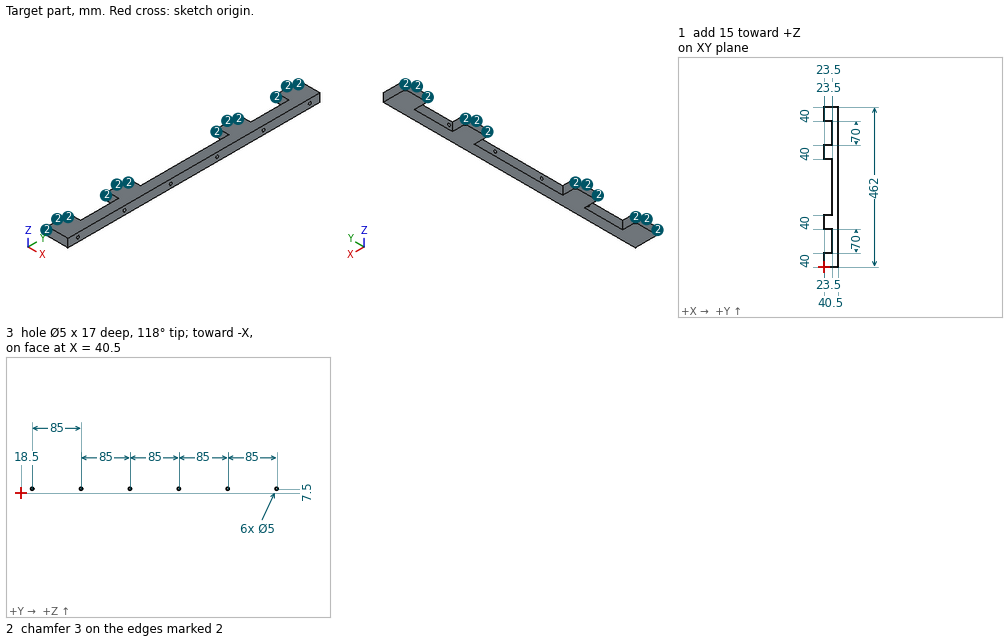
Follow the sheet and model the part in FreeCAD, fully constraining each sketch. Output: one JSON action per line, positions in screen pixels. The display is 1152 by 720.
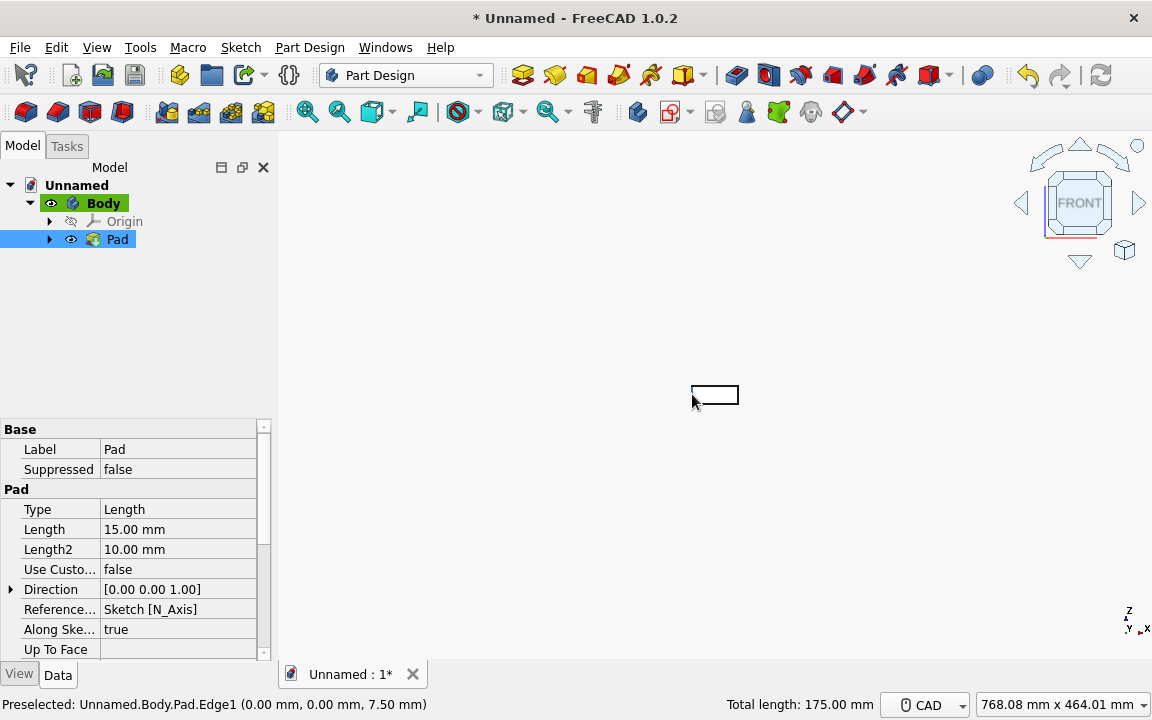
{"action": "scroll", "coordinate": [692, 394], "scroll_direction": "up", "scroll_amount": 5}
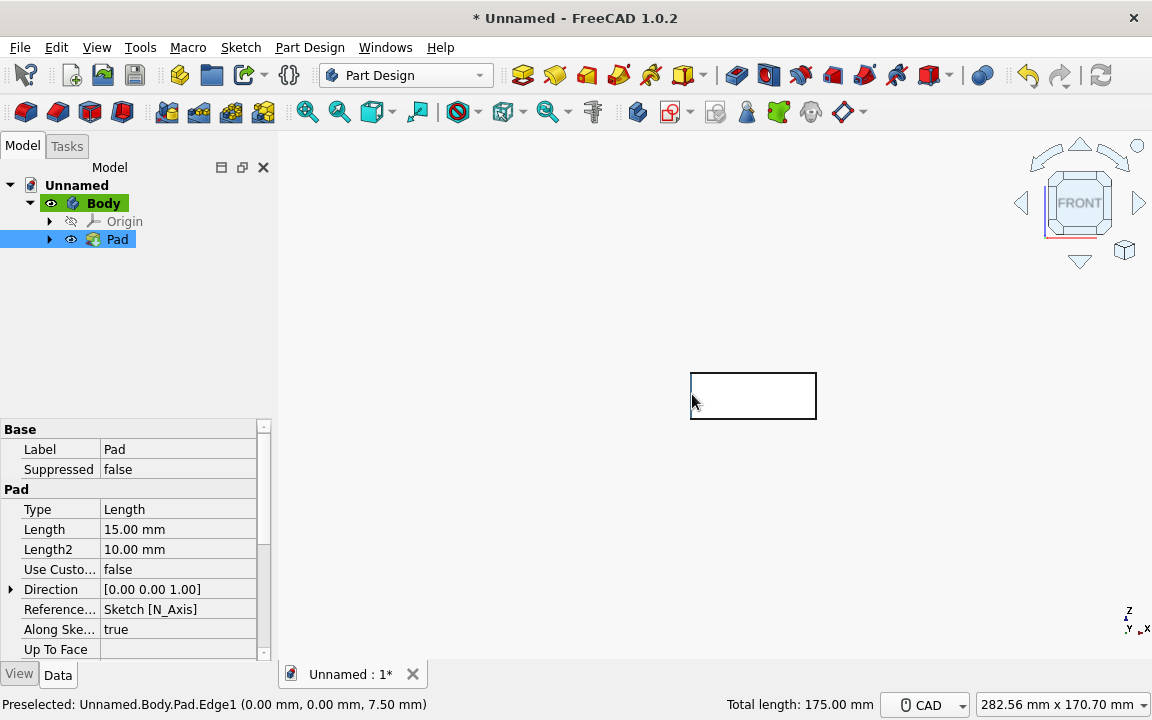
{"action": "left_click", "coordinate": [308, 112]}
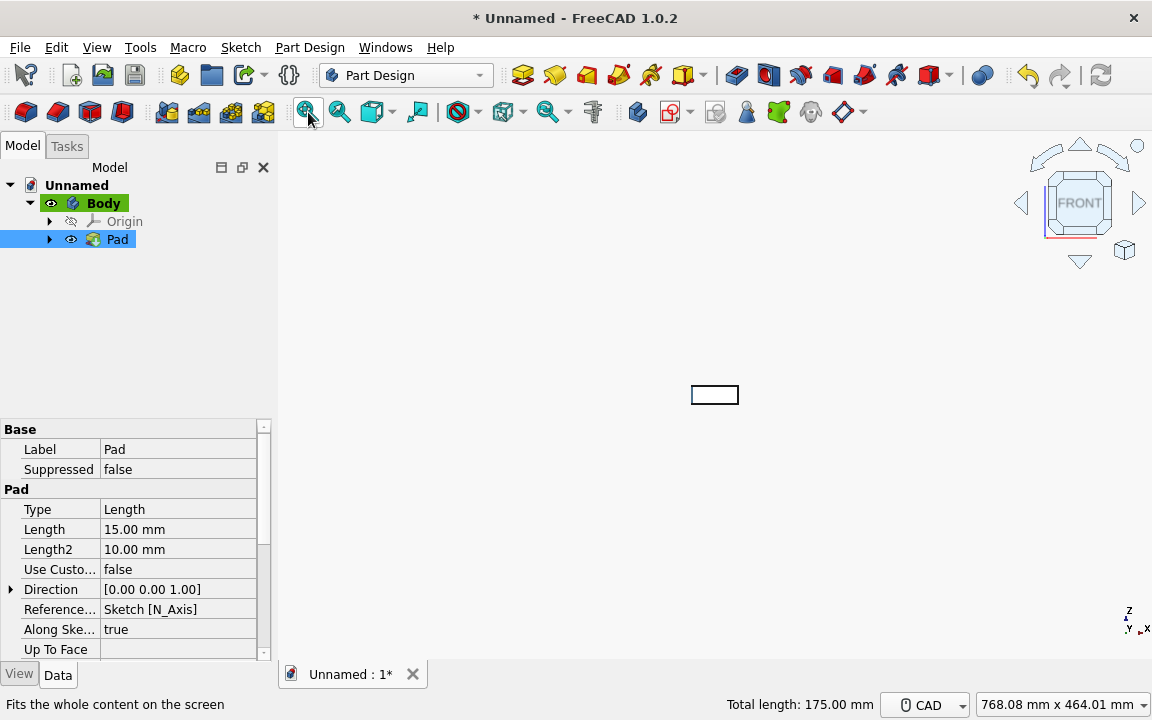
{"action": "key", "text": "3"}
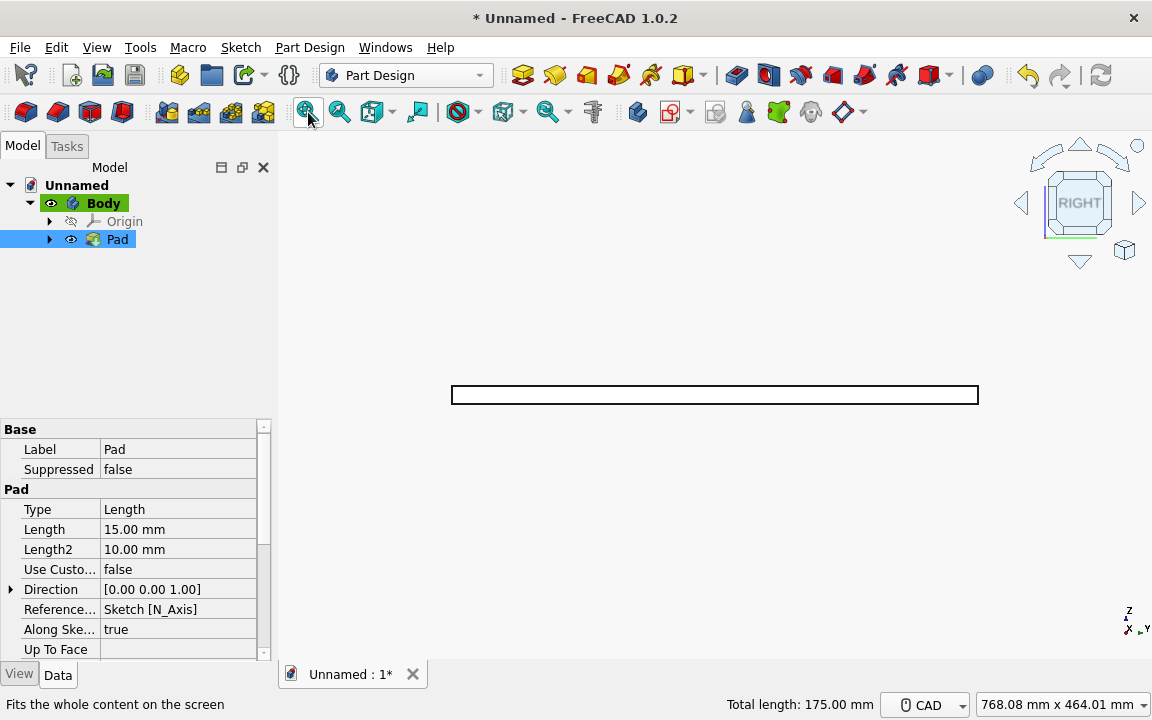
{"action": "scroll", "coordinate": [577, 394], "scroll_direction": "up", "scroll_amount": 5}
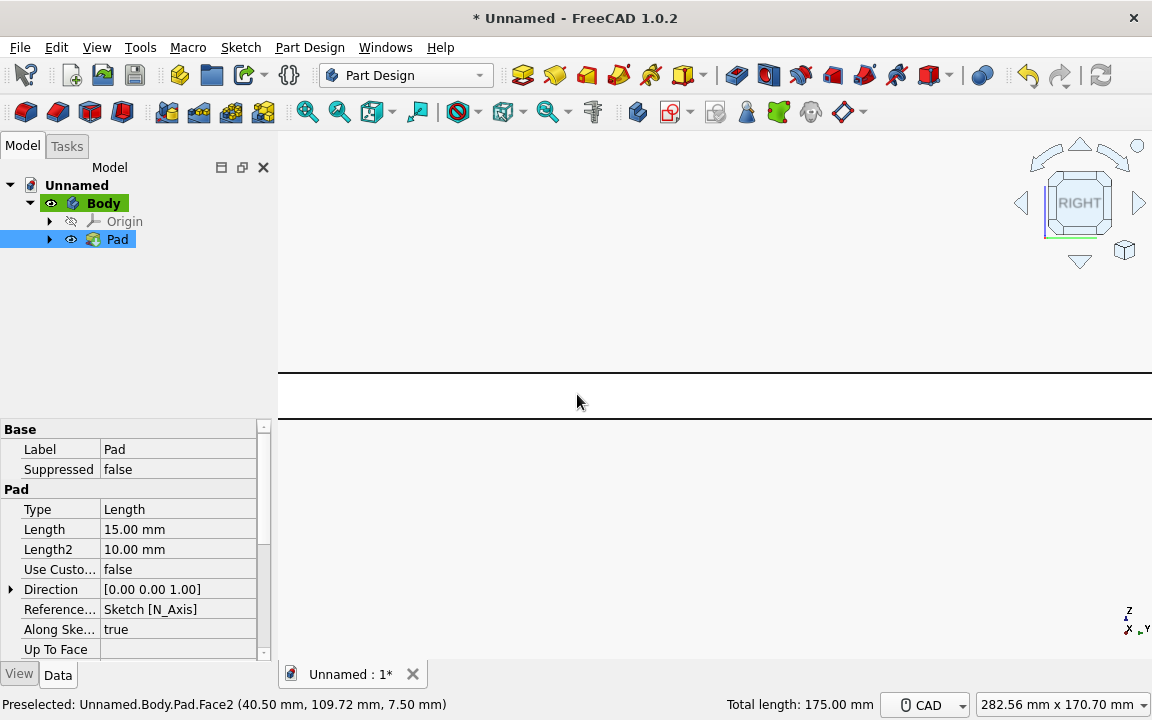
{"action": "left_click", "coordinate": [308, 112]}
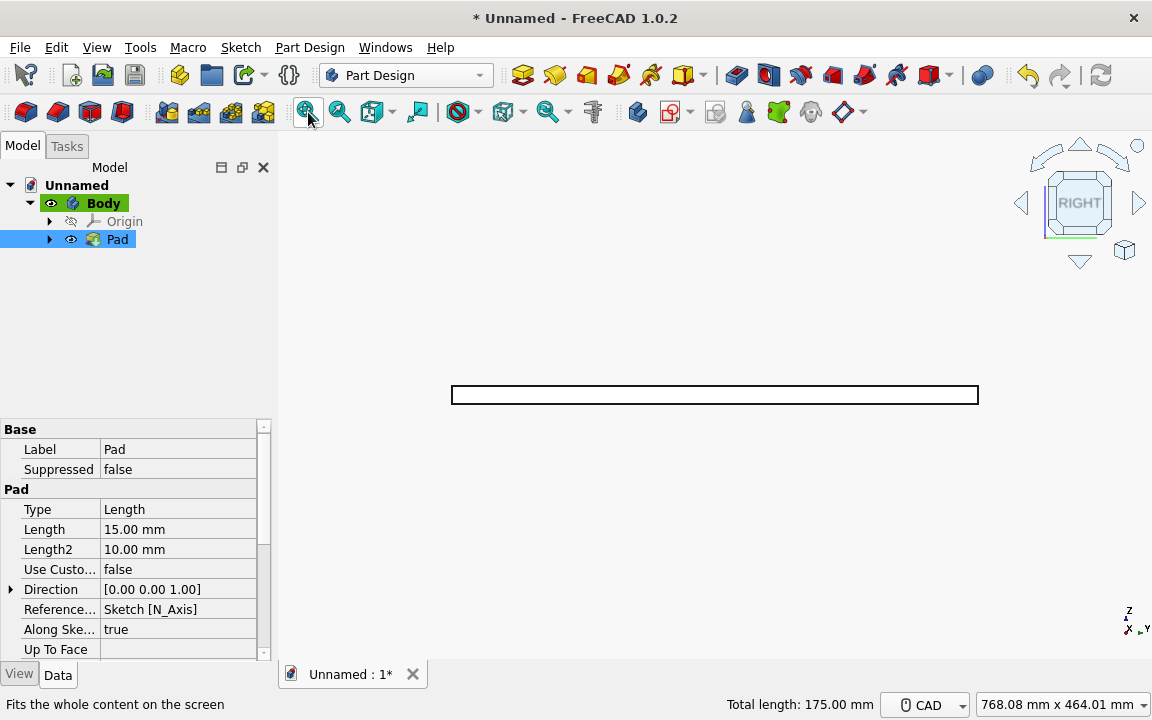
{"action": "key", "text": "5"}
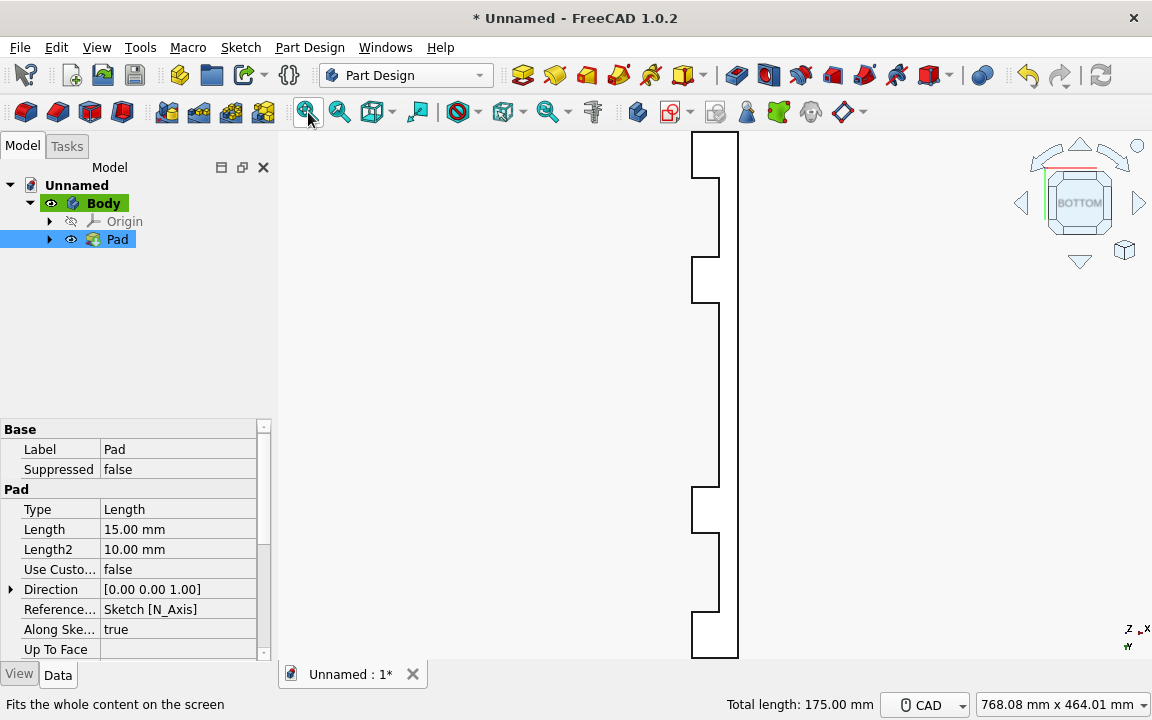
{"action": "scroll", "coordinate": [692, 256], "scroll_direction": "up", "scroll_amount": 5}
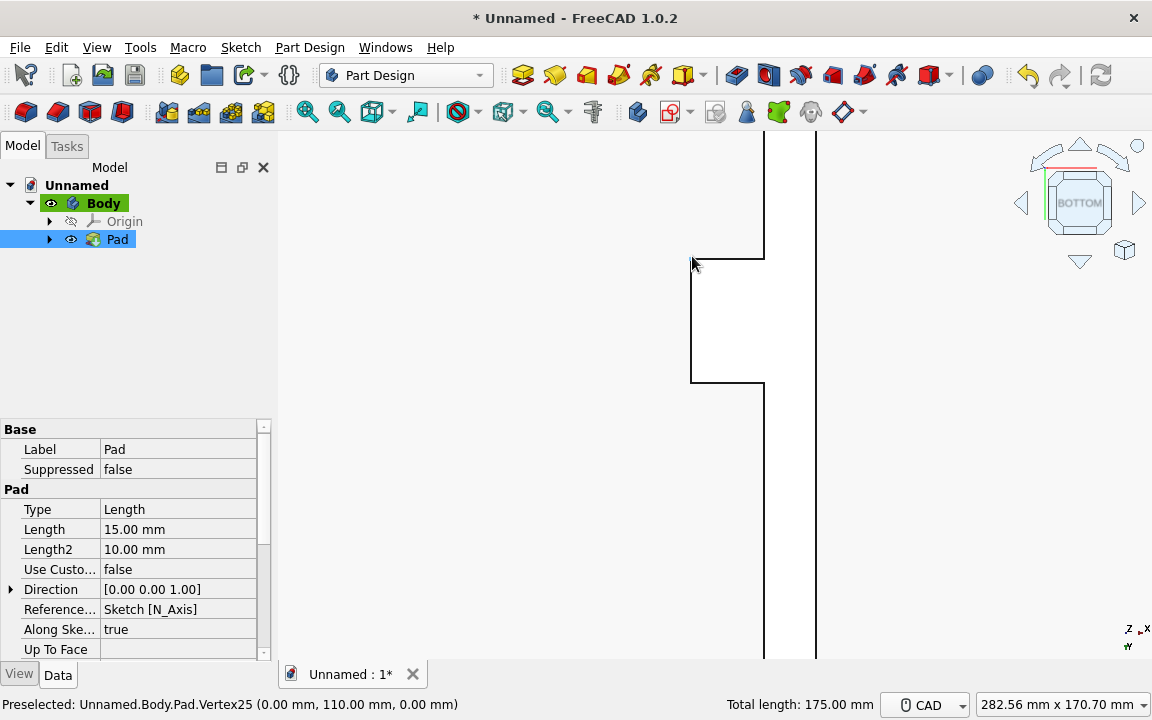
{"action": "key", "text": "v f"}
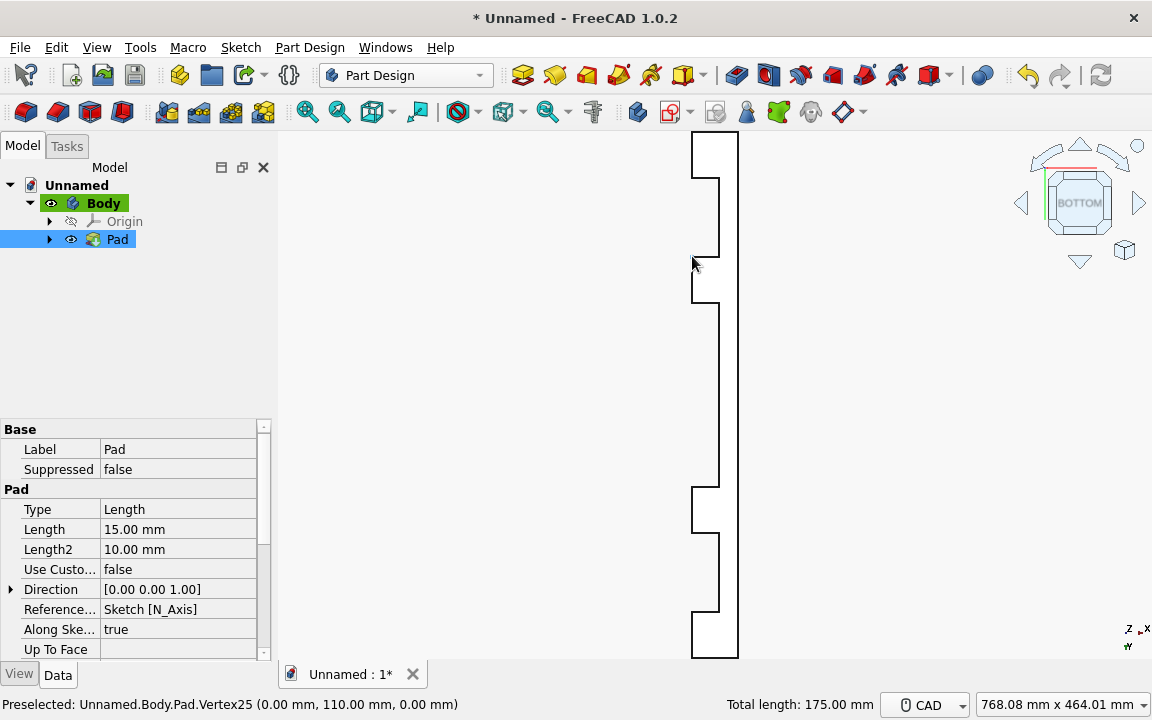
{"action": "key", "text": "4"}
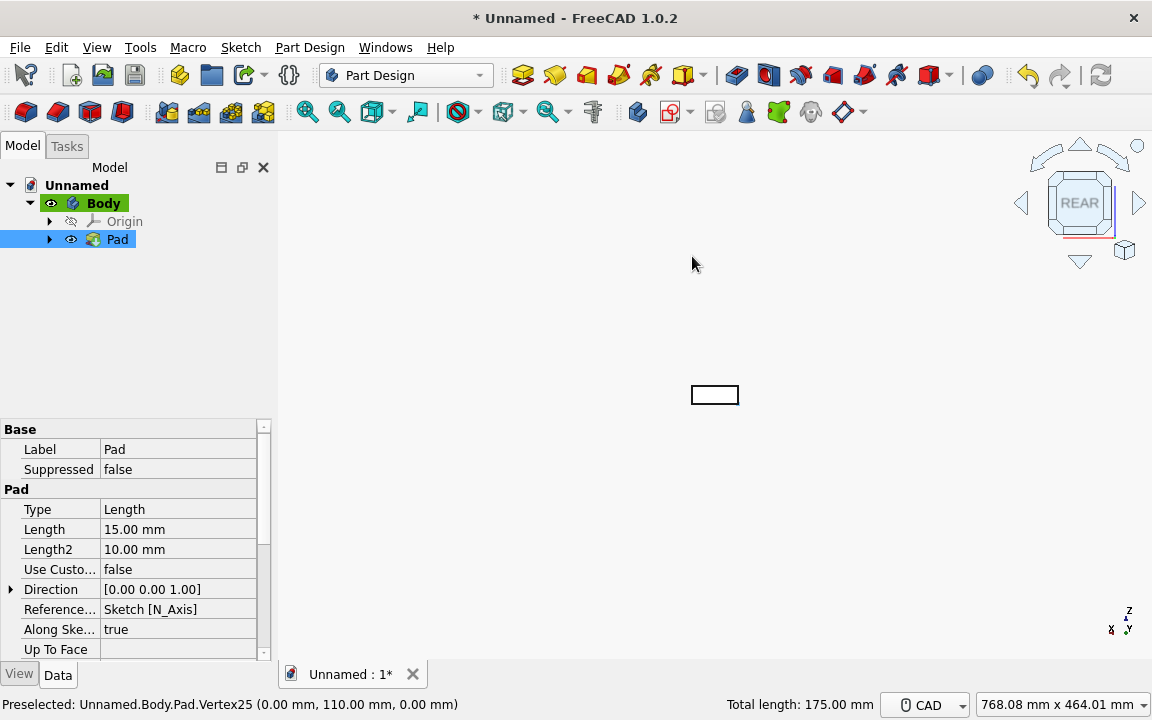
{"action": "left_click", "coordinate": [308, 112]}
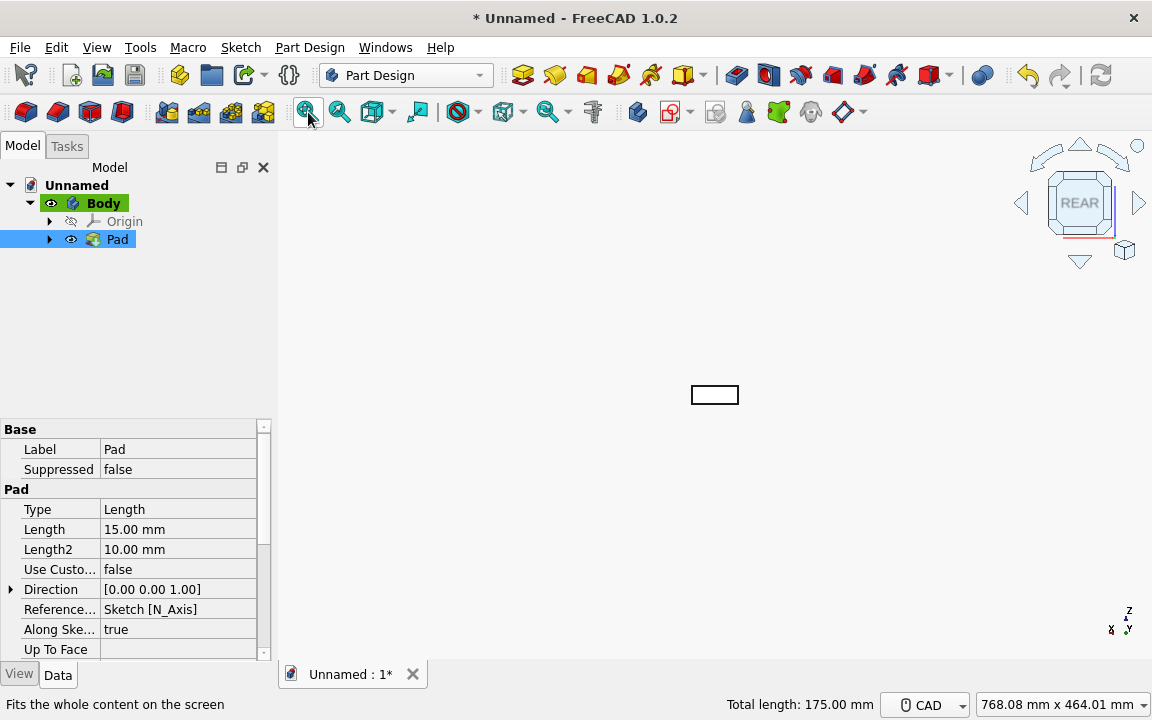
{"action": "left_click", "coordinate": [738, 394], "text": "ctrl"}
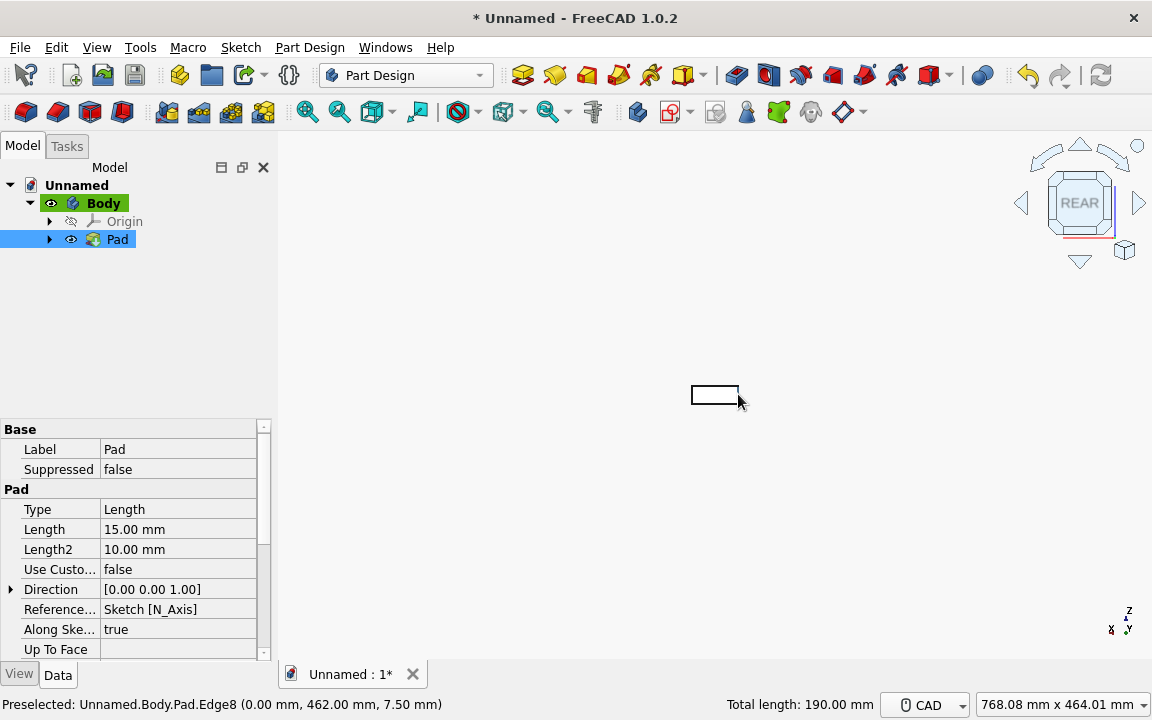
{"action": "scroll", "coordinate": [738, 394], "scroll_direction": "up", "scroll_amount": 5}